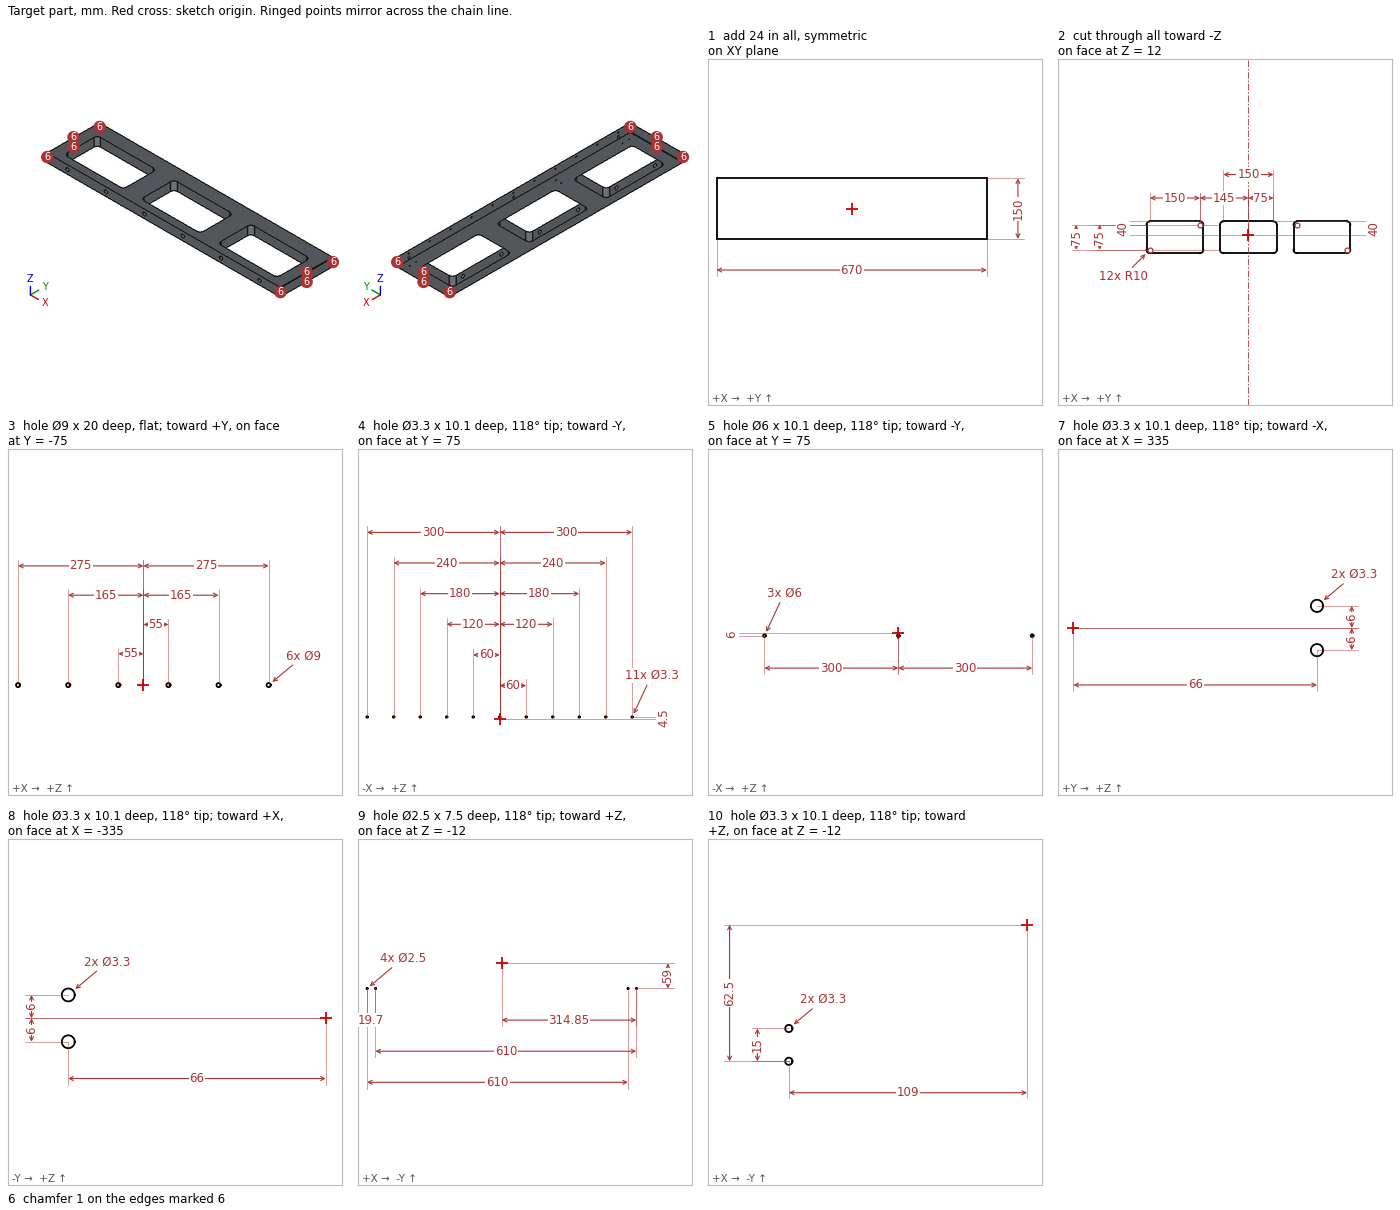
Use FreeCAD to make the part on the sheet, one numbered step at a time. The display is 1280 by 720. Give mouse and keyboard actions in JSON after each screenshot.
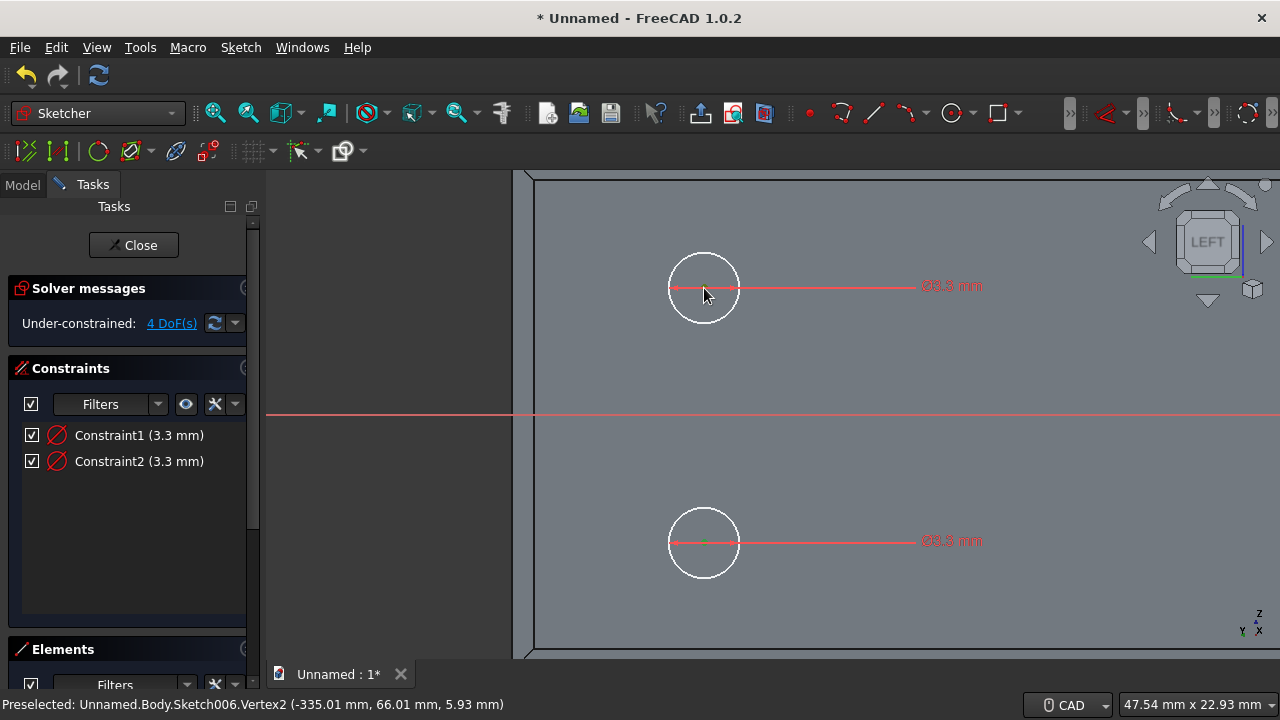
{"action": "key", "text": "v"}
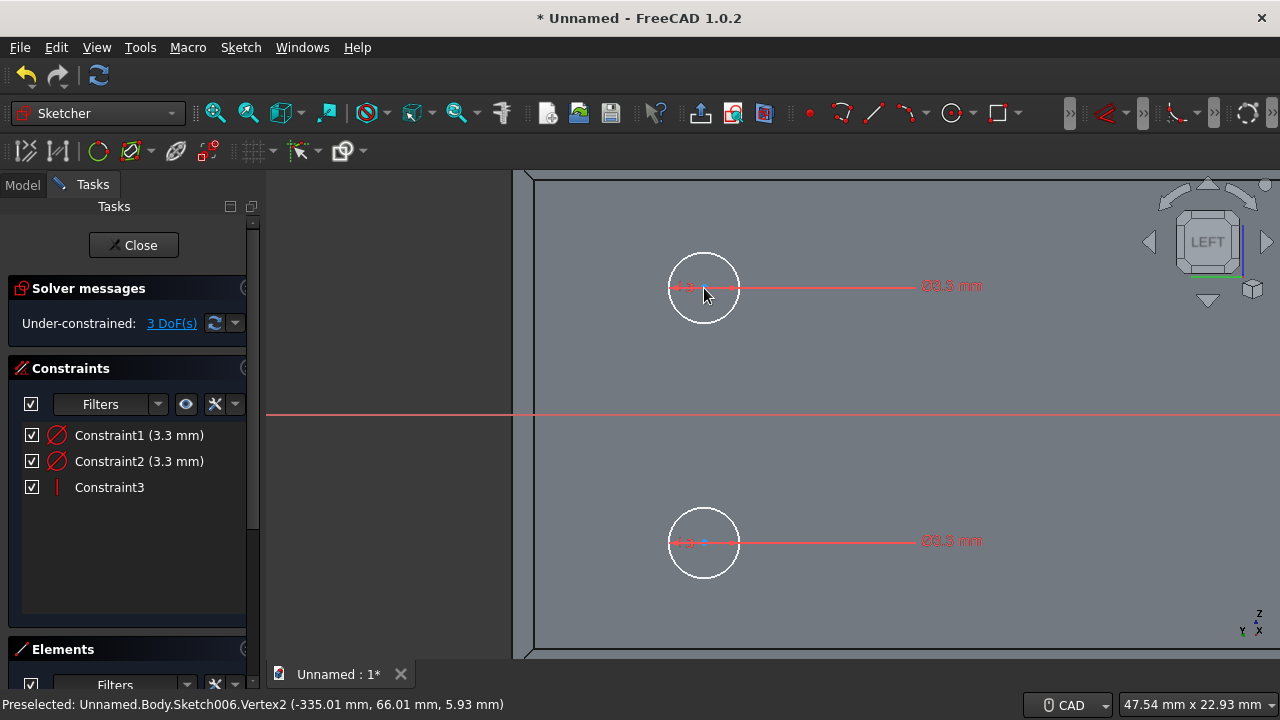
{"action": "key", "text": "d"}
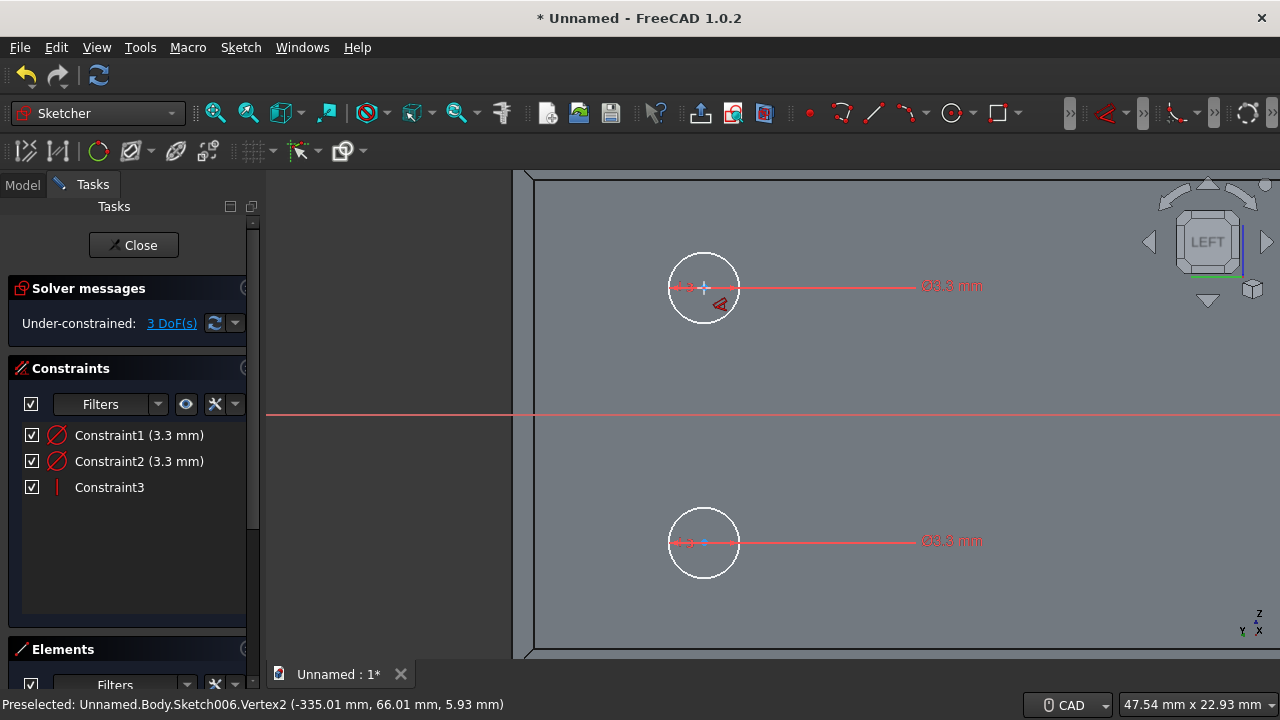
{"action": "left_click", "coordinate": [704, 543]}
{"action": "left_click", "coordinate": [670, 479]}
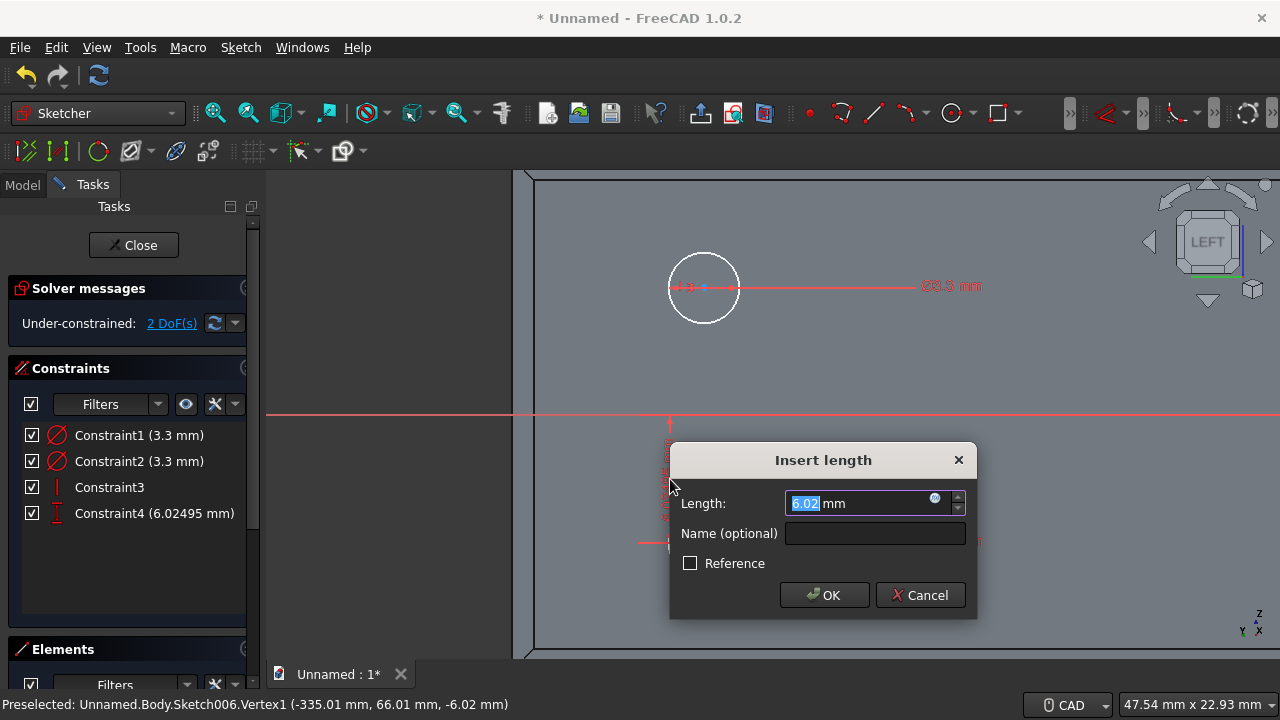
{"action": "type", "text": "6"}
{"action": "key", "text": "Return"}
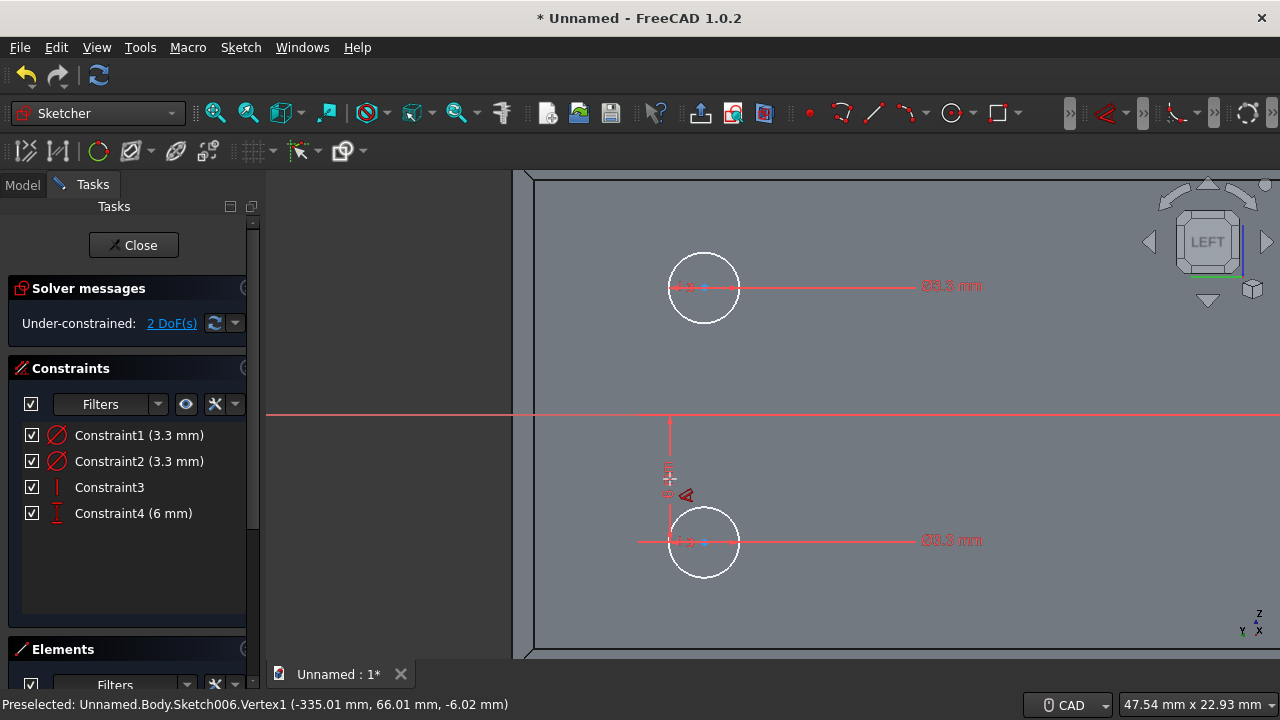
{"action": "left_click", "coordinate": [704, 288]}
{"action": "left_click", "coordinate": [670, 351]}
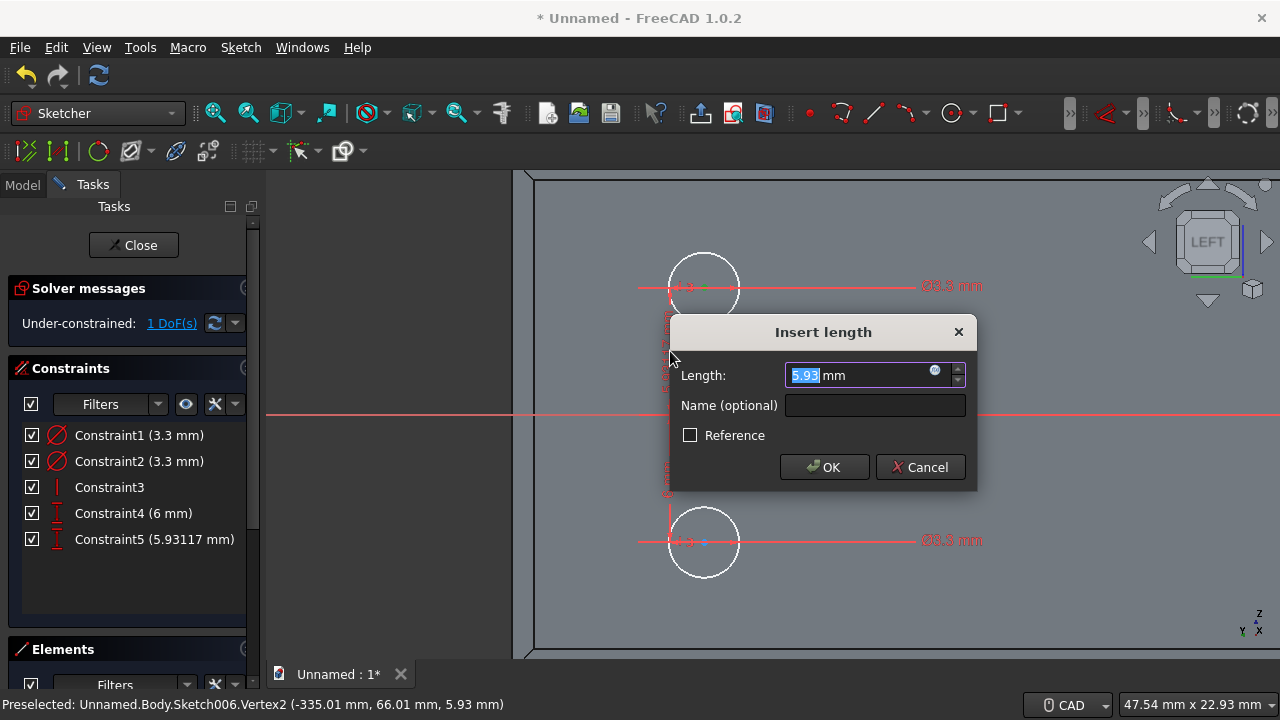
{"action": "type", "text": "6"}
{"action": "key", "text": "Return"}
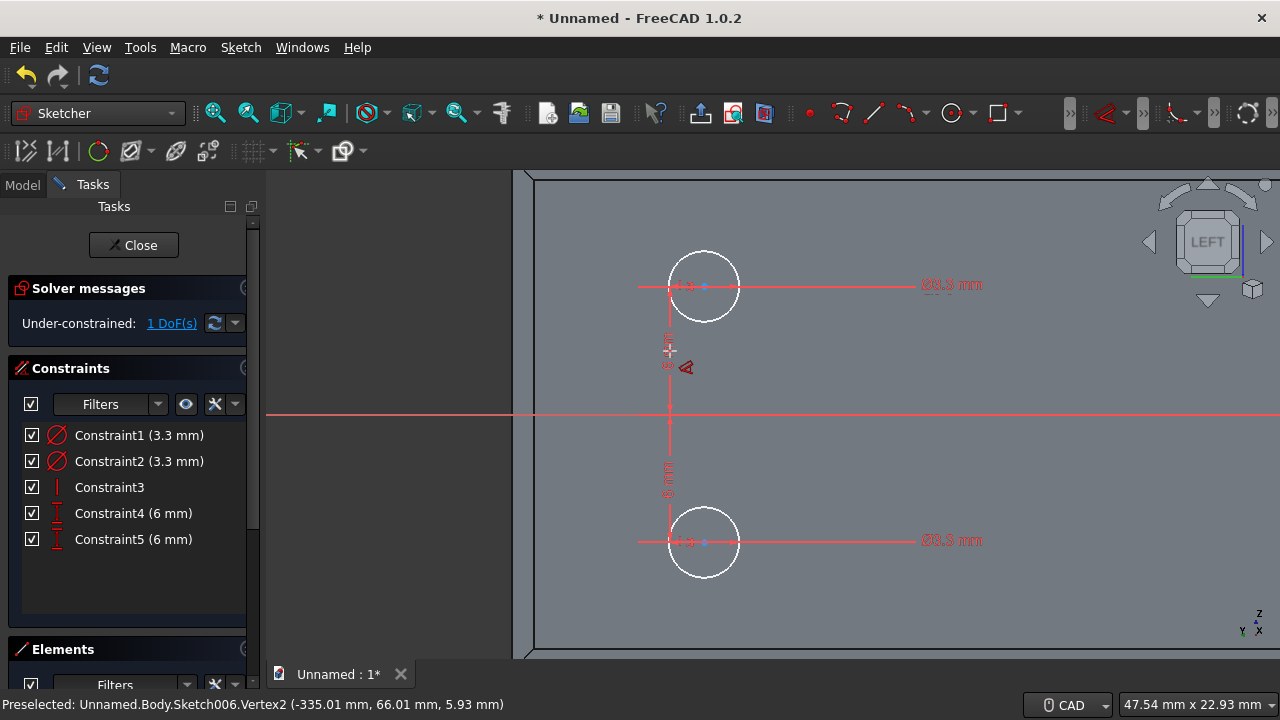
{"action": "left_click", "coordinate": [704, 542]}
{"action": "left_click", "coordinate": [910, 576]}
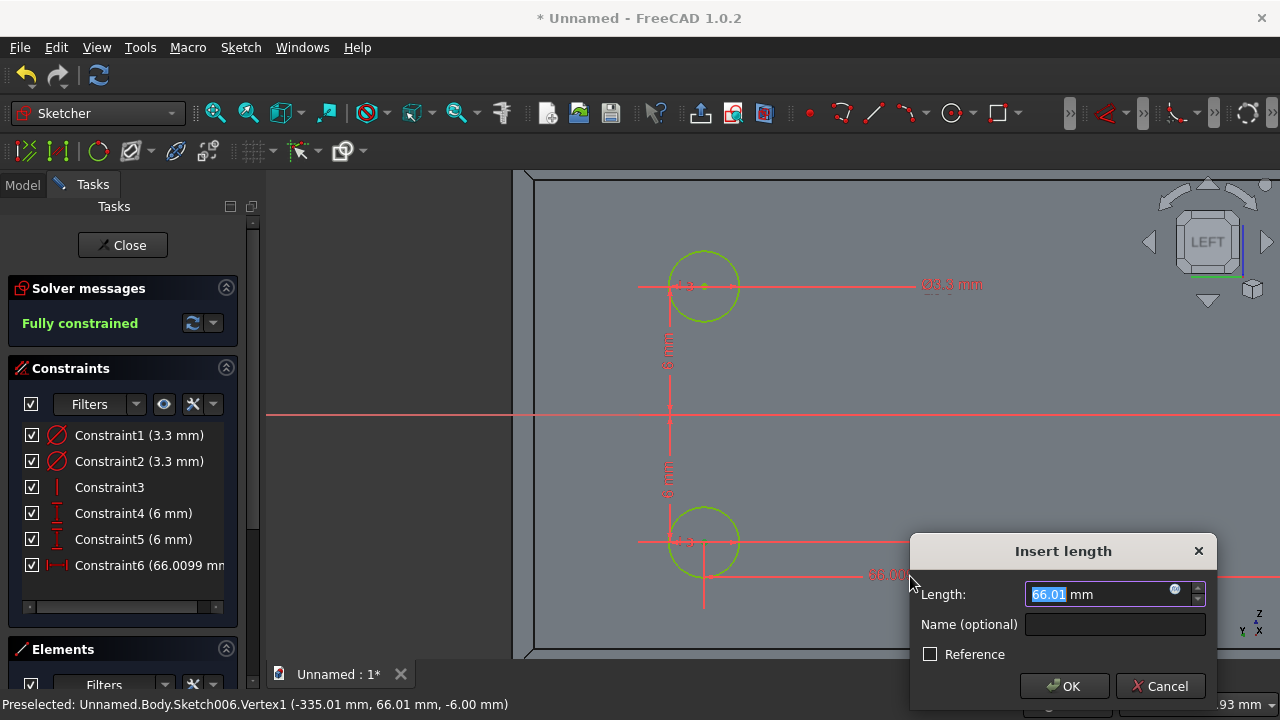
{"action": "type", "text": "66"}
{"action": "key", "text": "Return"}
{"action": "key", "text": "Escape"}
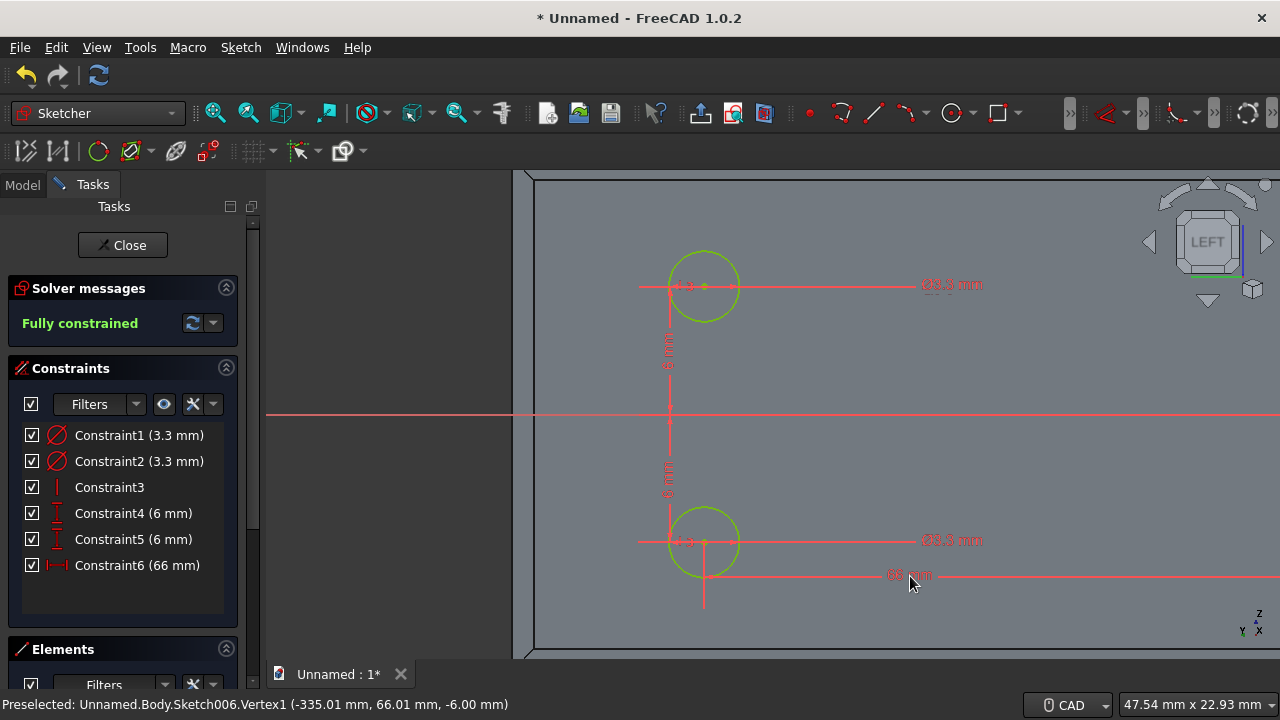
{"action": "left_click", "coordinate": [123, 245]}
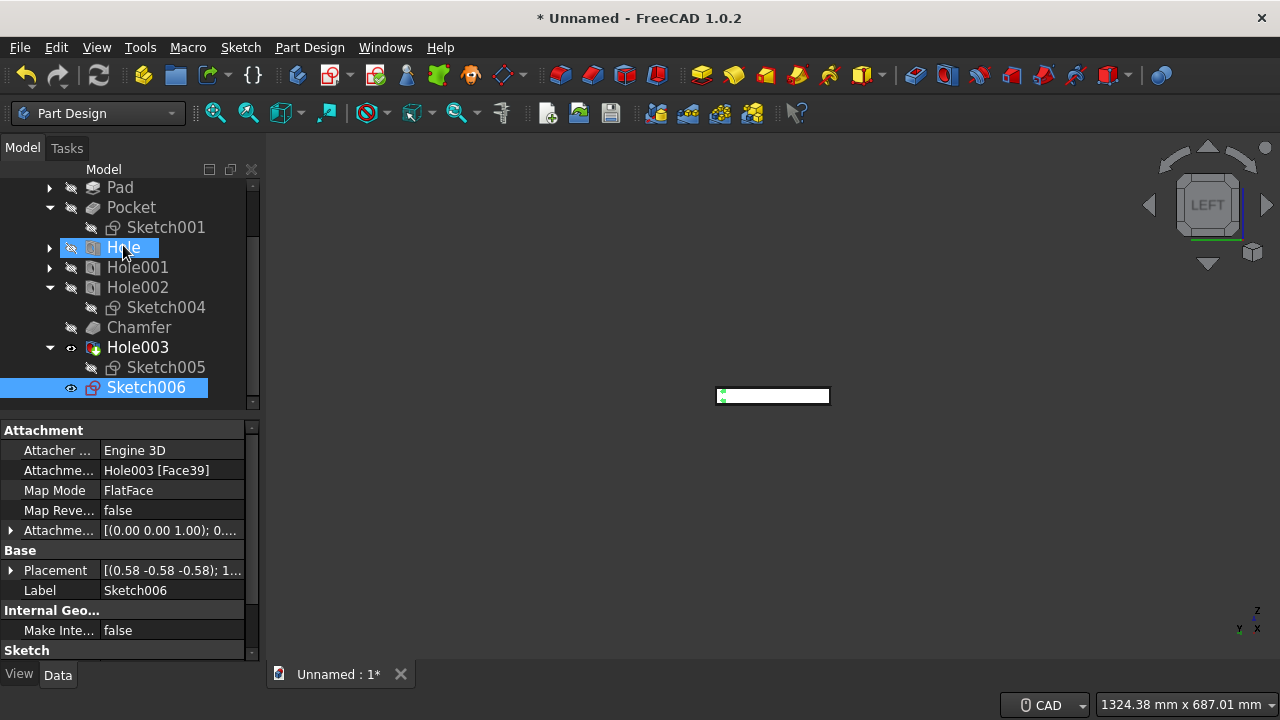
{"action": "left_click", "coordinate": [948, 76]}